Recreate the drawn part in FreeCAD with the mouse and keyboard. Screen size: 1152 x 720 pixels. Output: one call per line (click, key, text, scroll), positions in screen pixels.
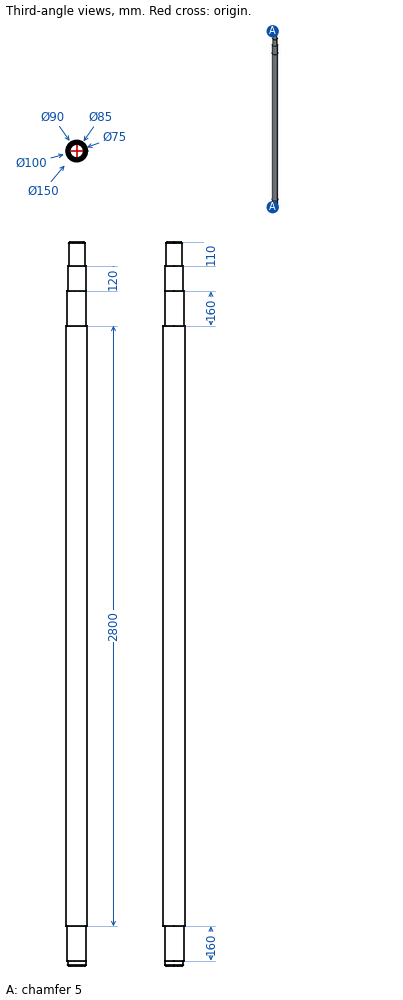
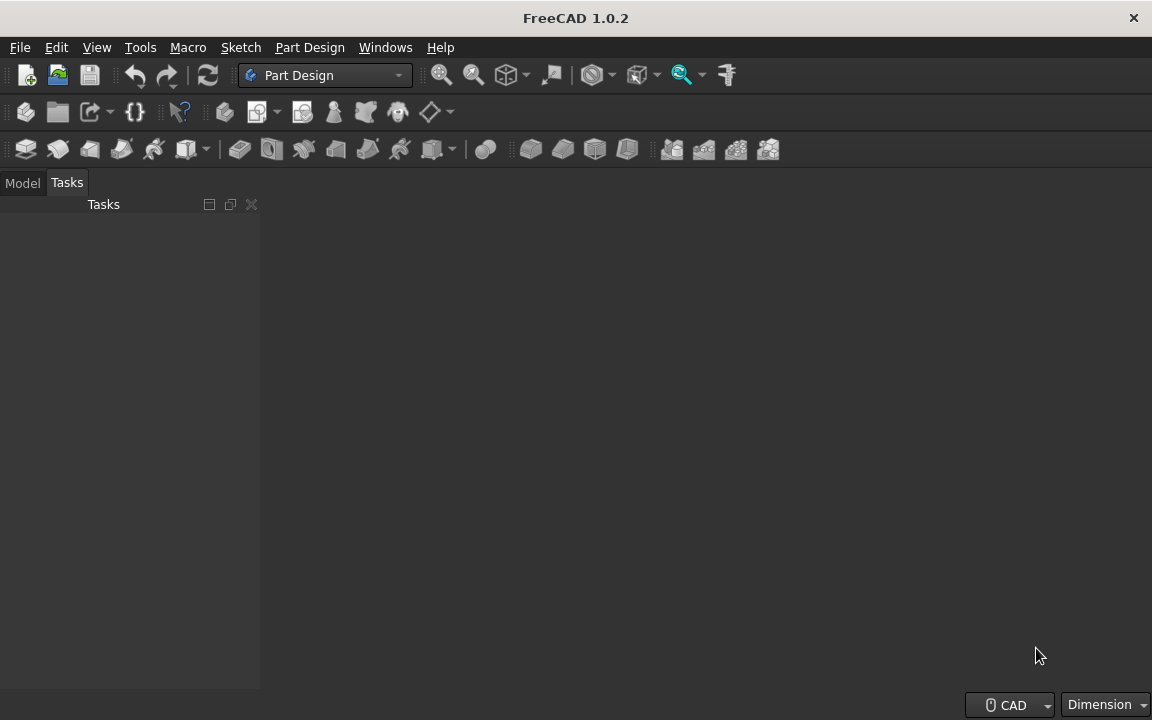
click(216, 150)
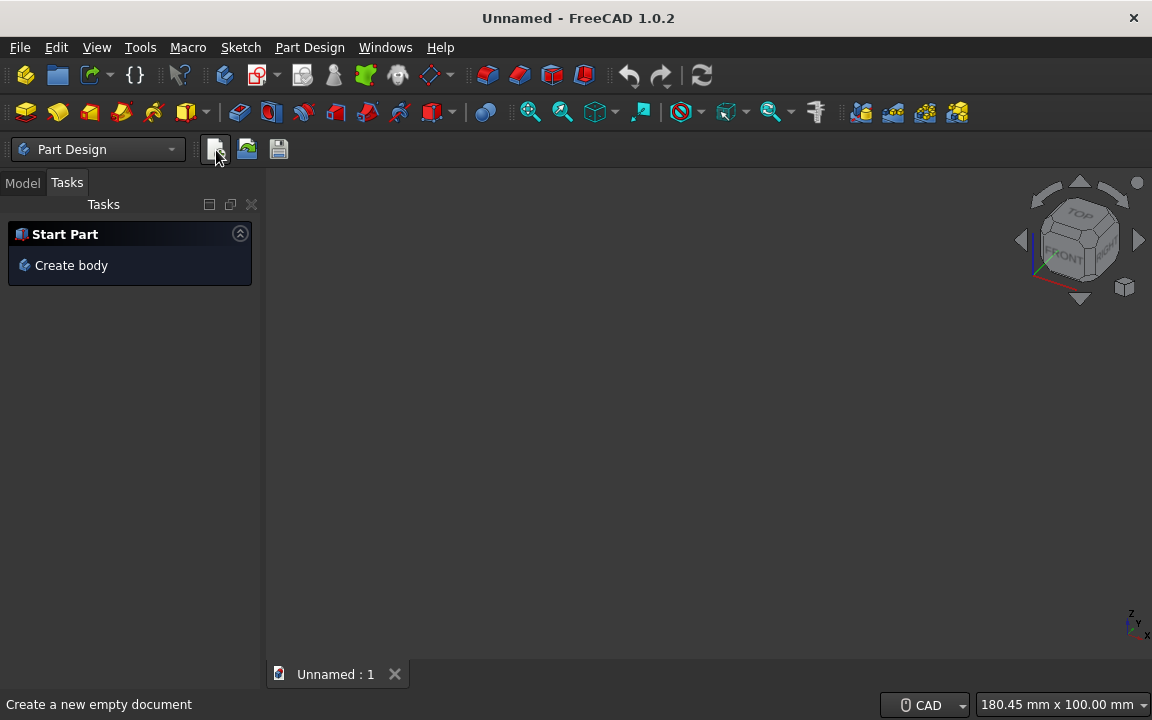
click(258, 76)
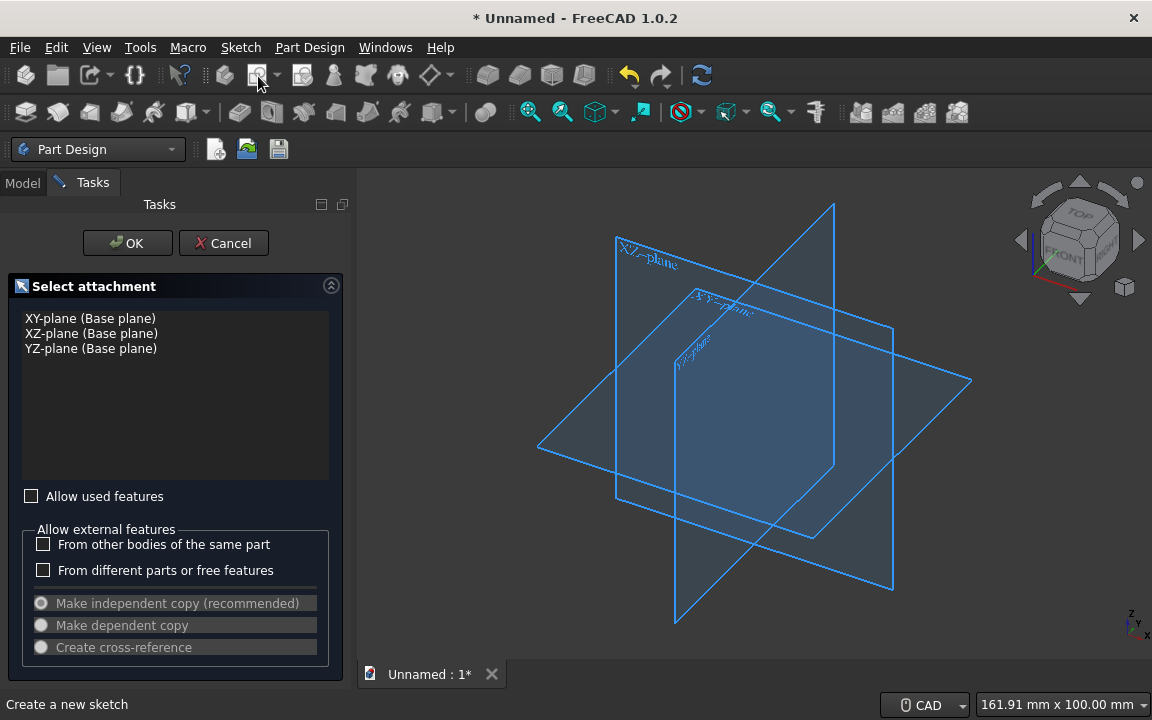
click(82, 318)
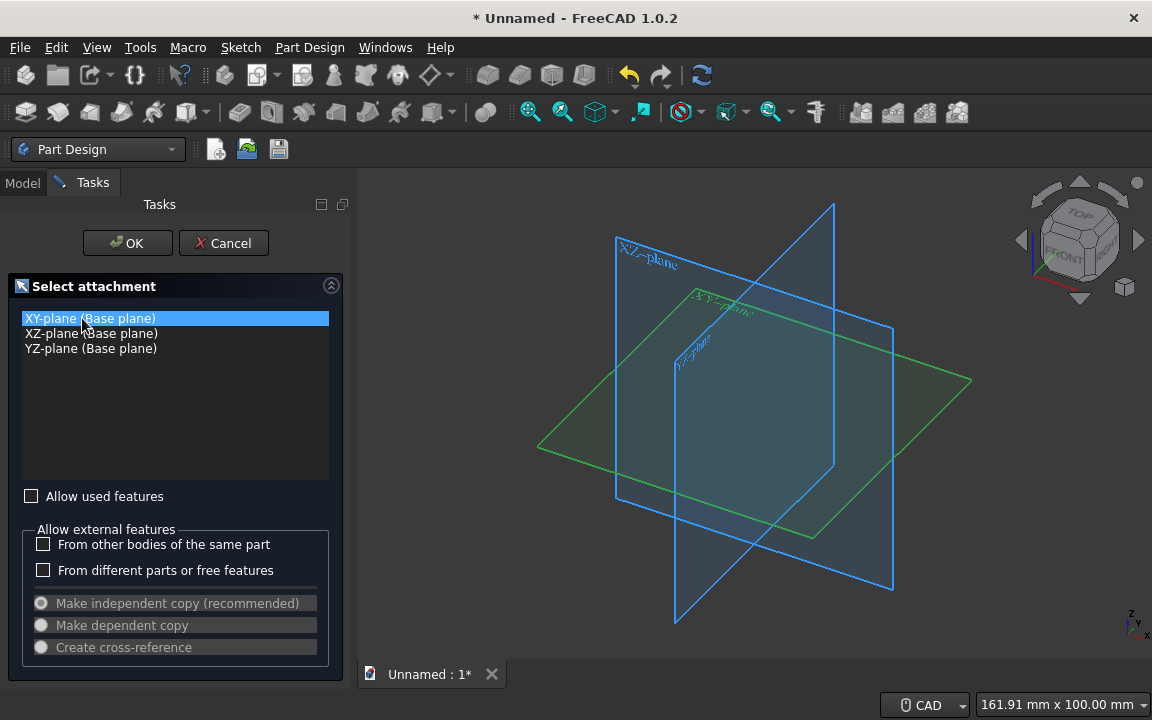
click(128, 243)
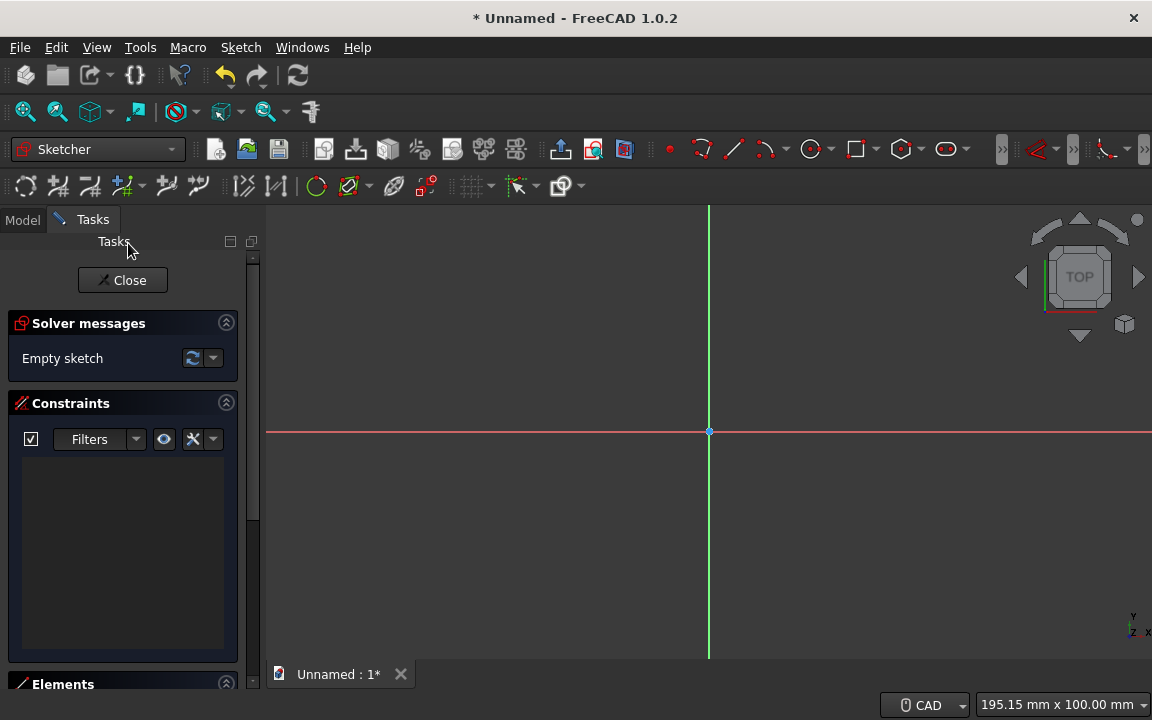
key(g)
key(c)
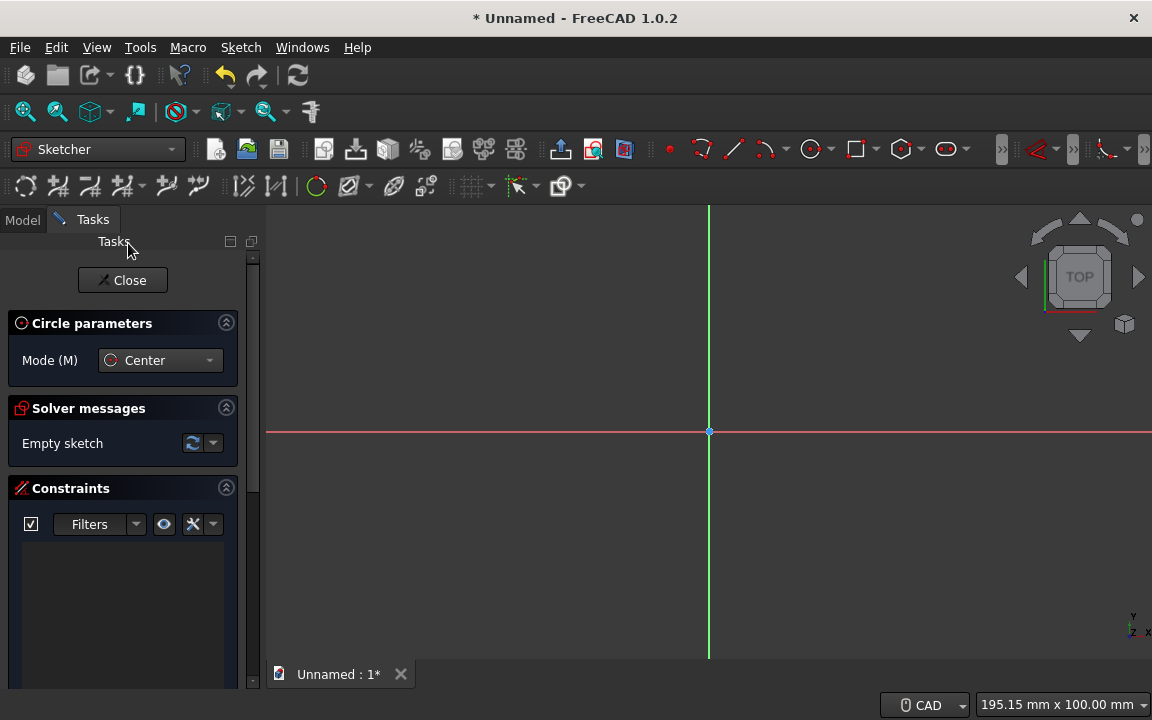
click(709, 432)
click(829, 312)
key(Escape)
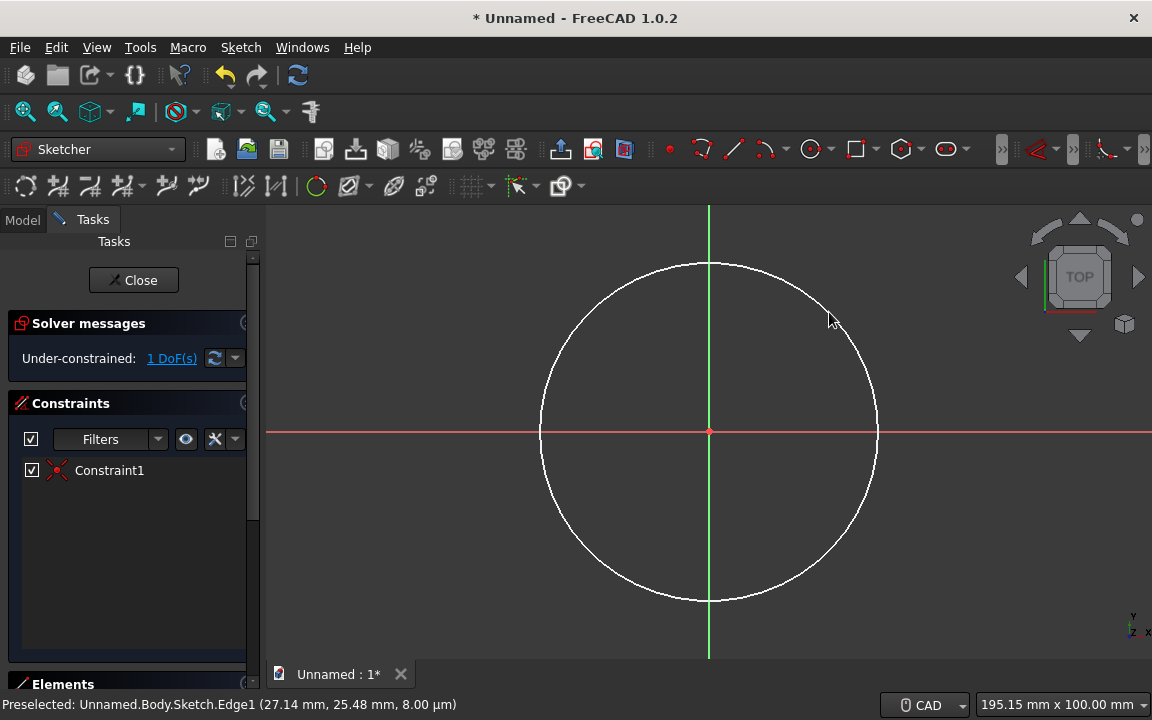
click(828, 312)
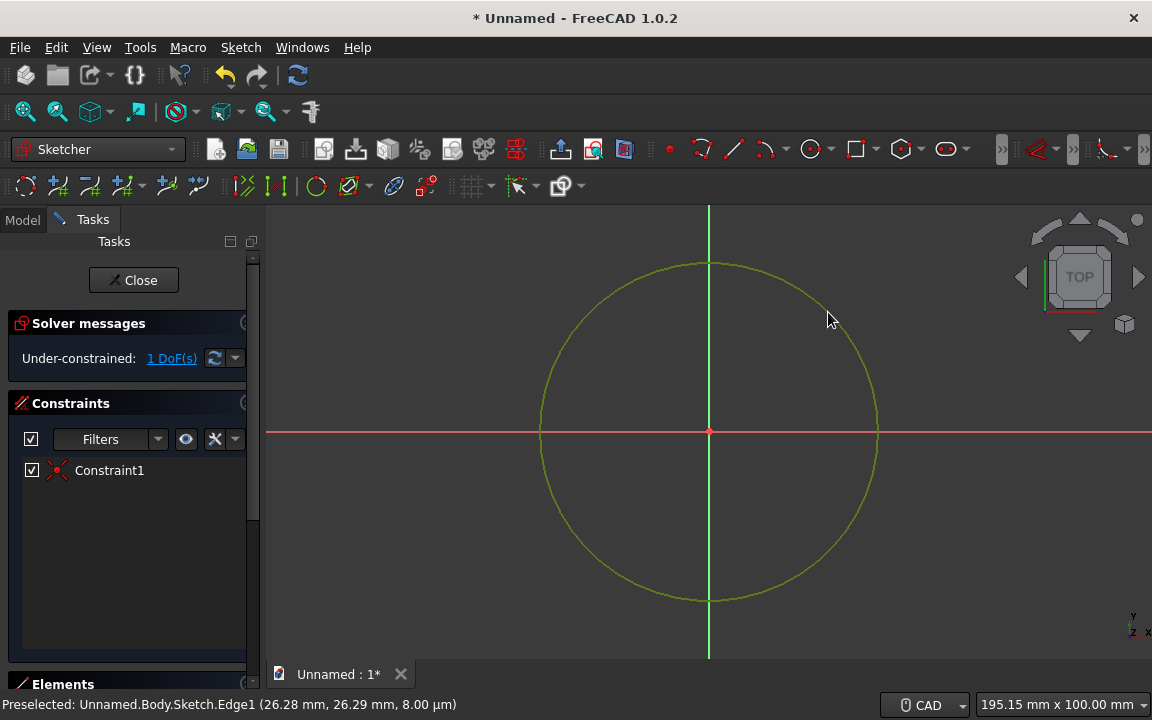
click(1058, 150)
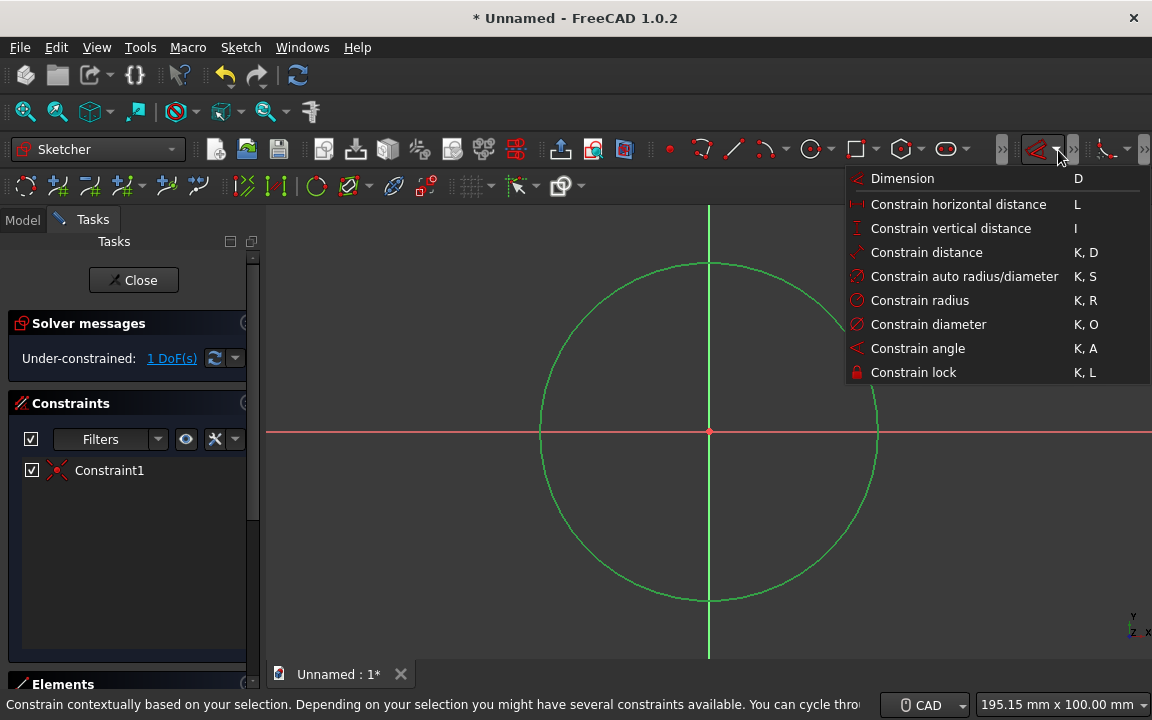
click(998, 324)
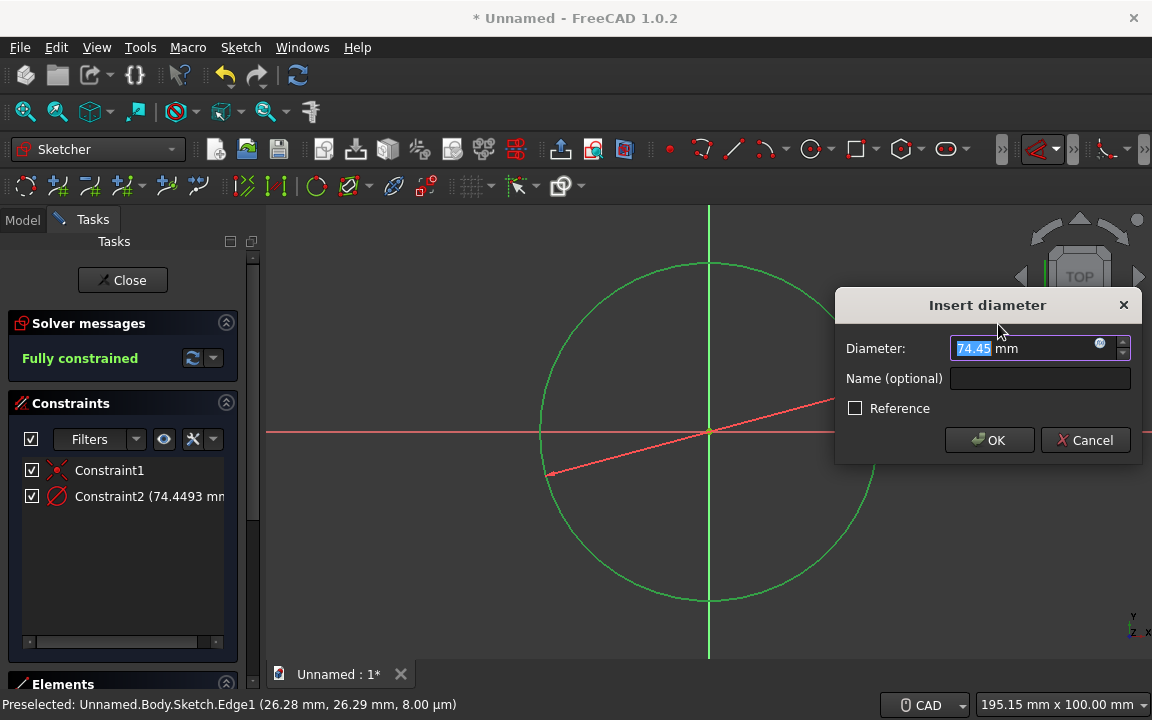
text(75)
key(Return)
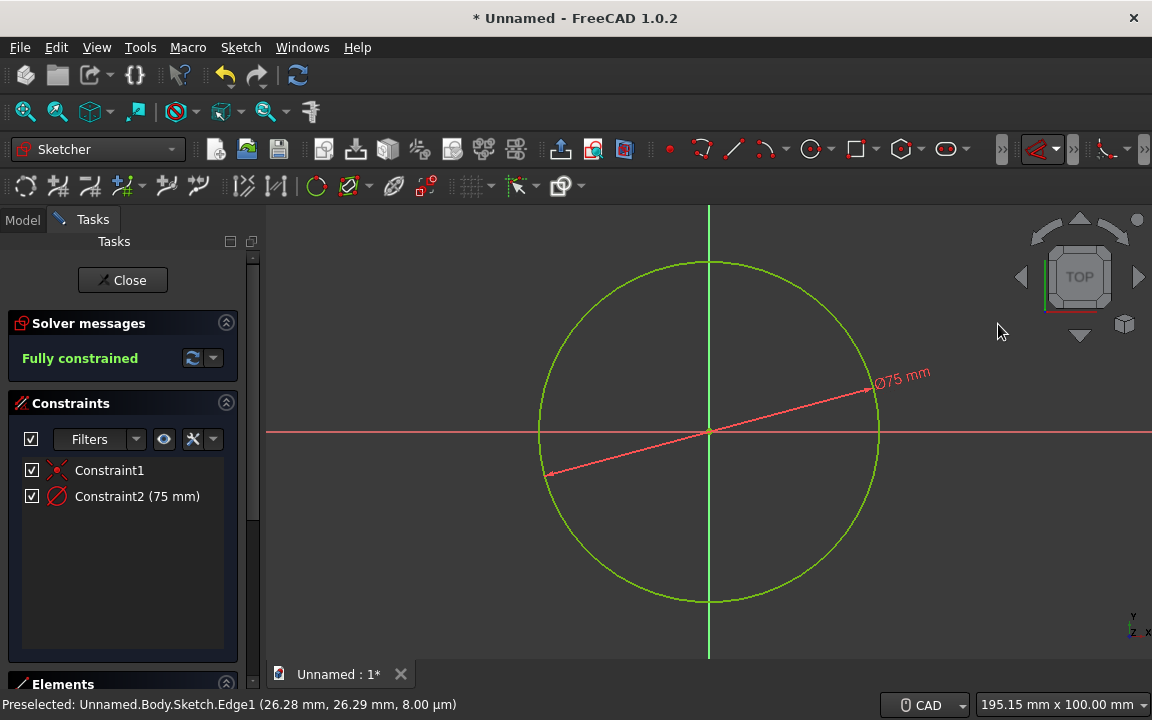
click(123, 280)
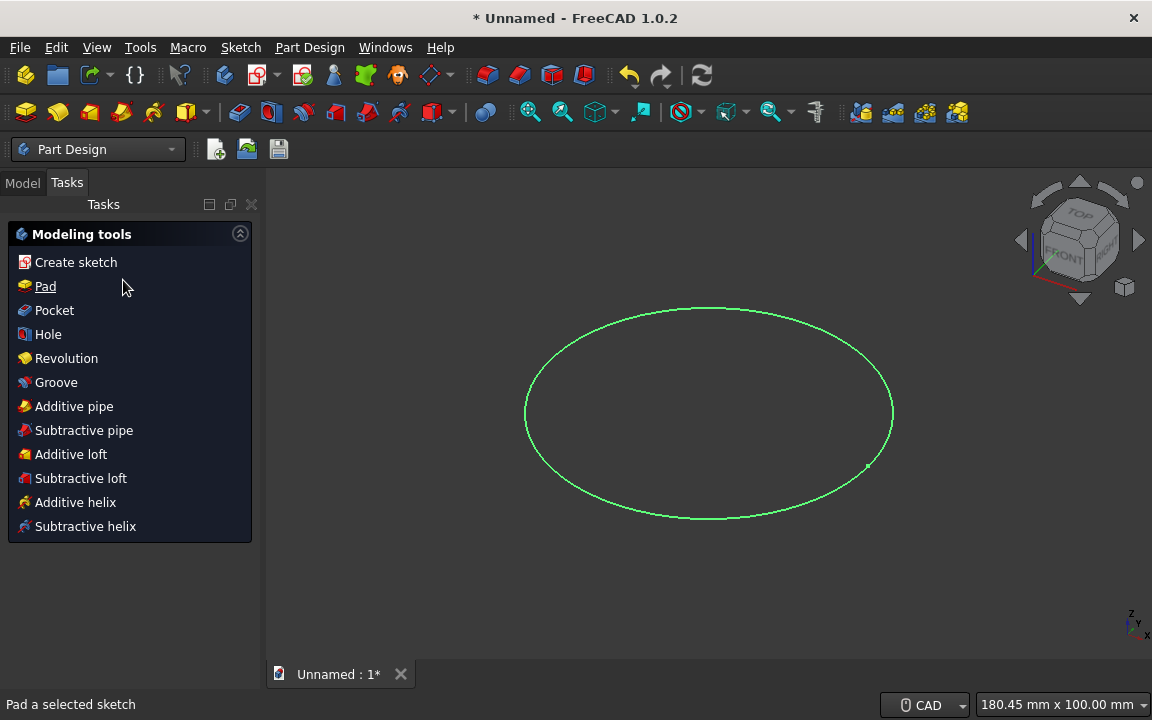
click(26, 112)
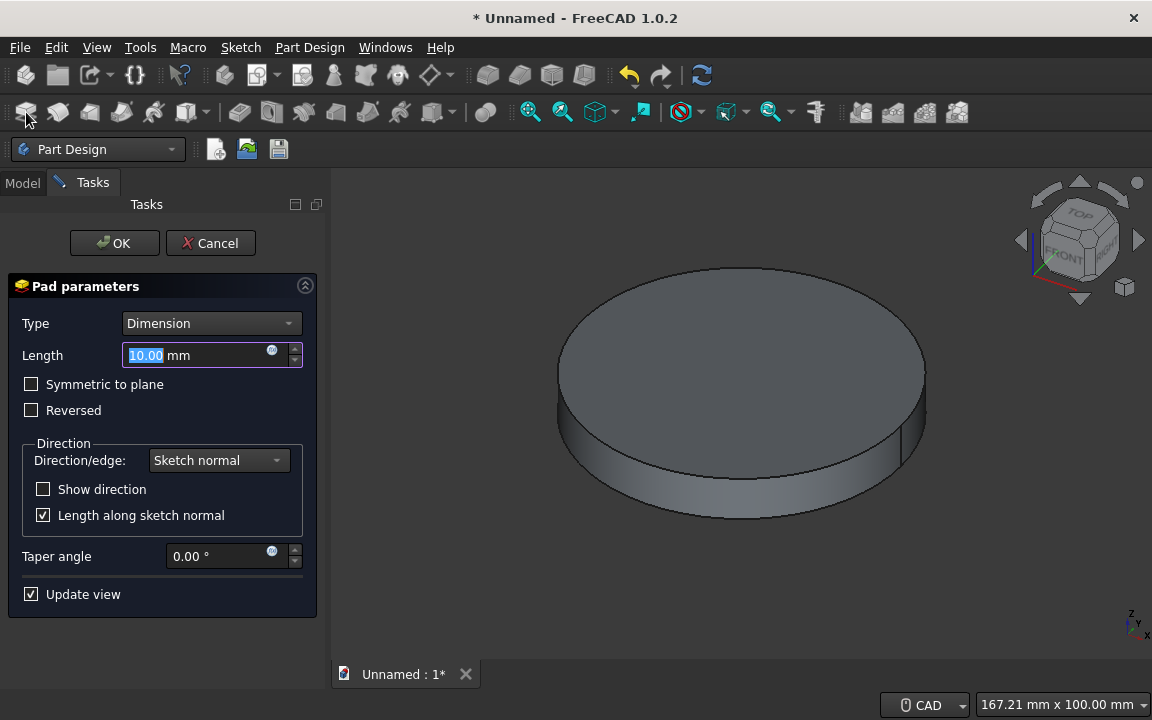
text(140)
key(Tab)